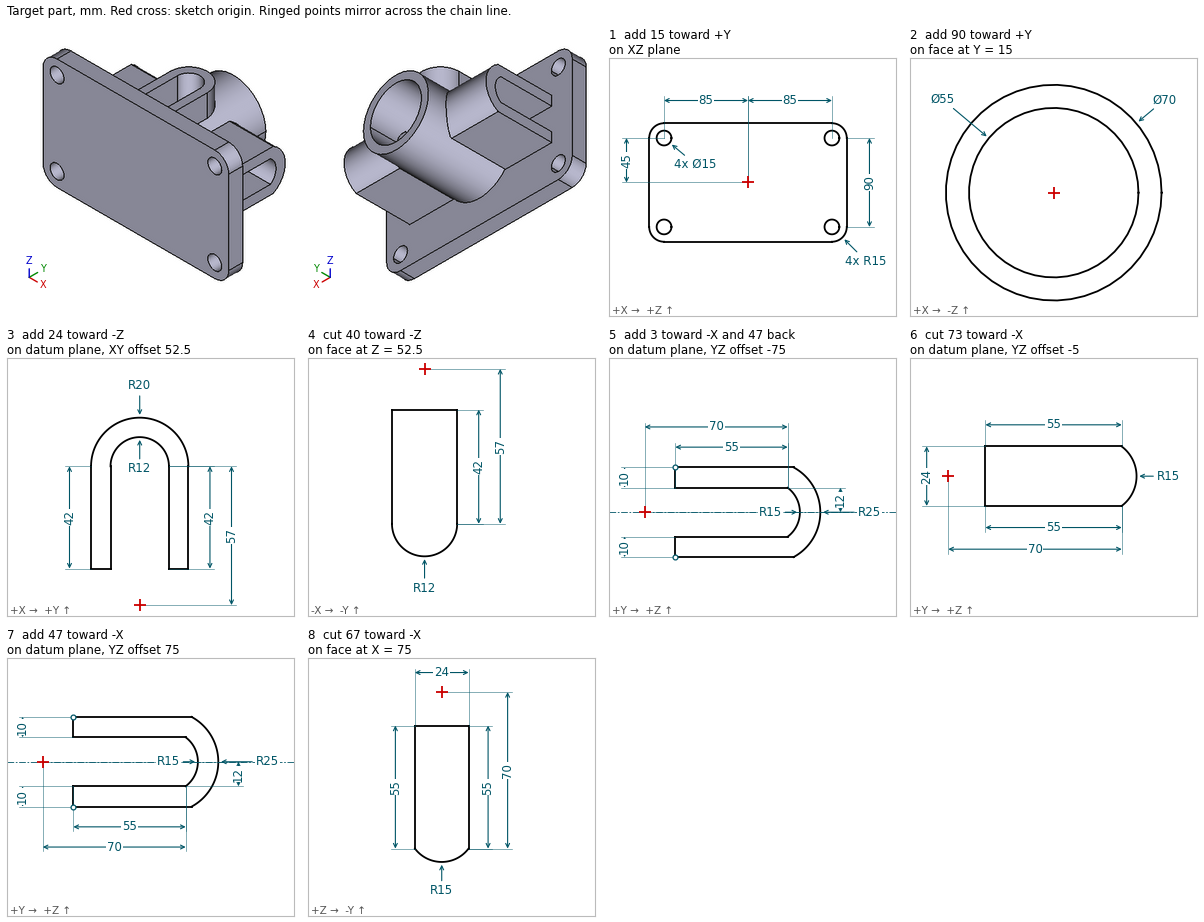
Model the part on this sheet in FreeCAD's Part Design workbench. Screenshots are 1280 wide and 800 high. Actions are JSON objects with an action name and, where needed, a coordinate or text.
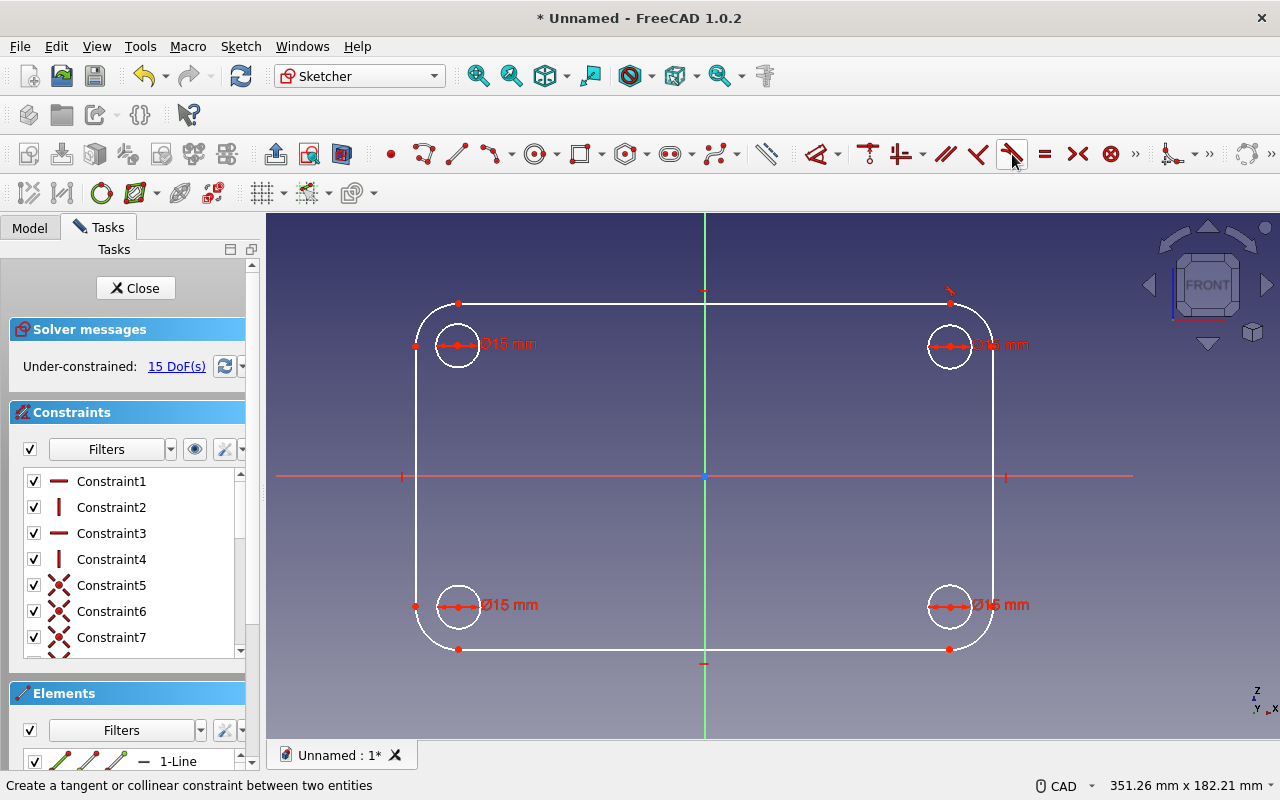
{"action": "left_click", "coordinate": [606, 304]}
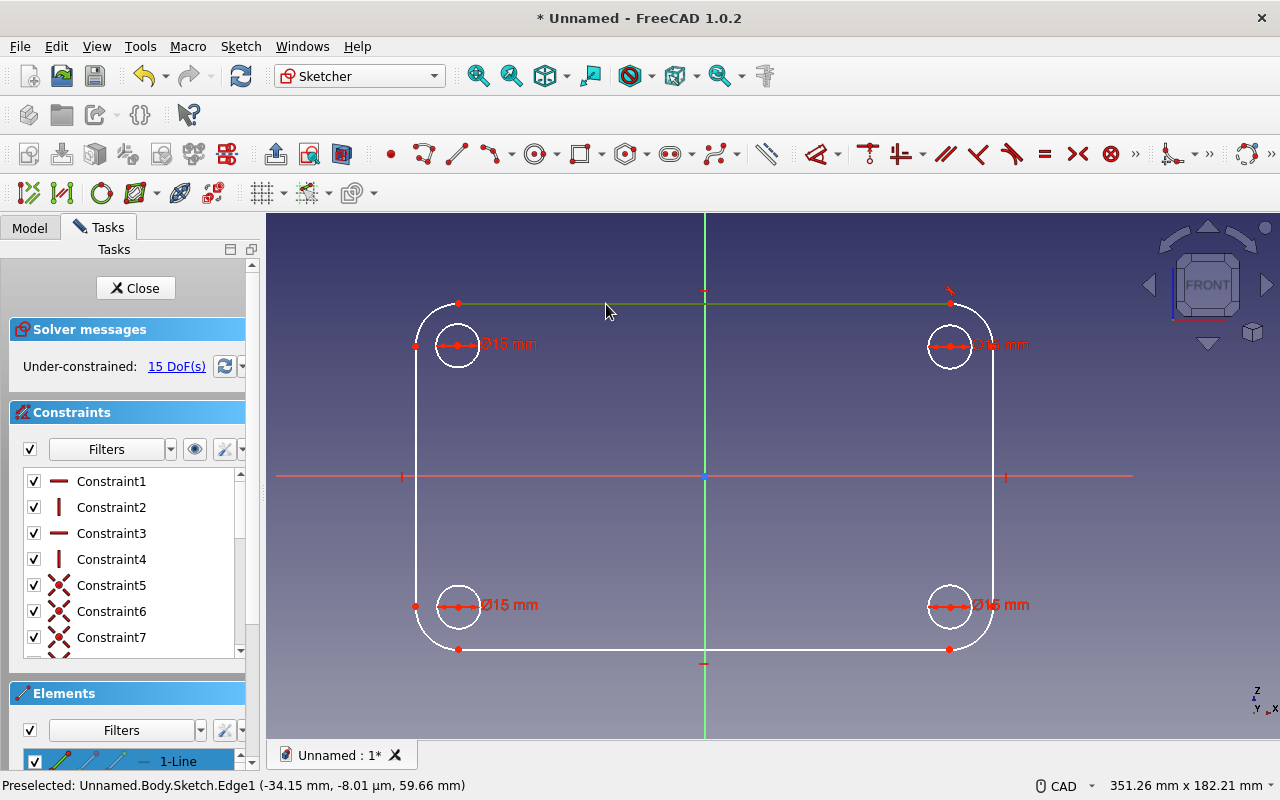
{"action": "left_click", "coordinate": [439, 308]}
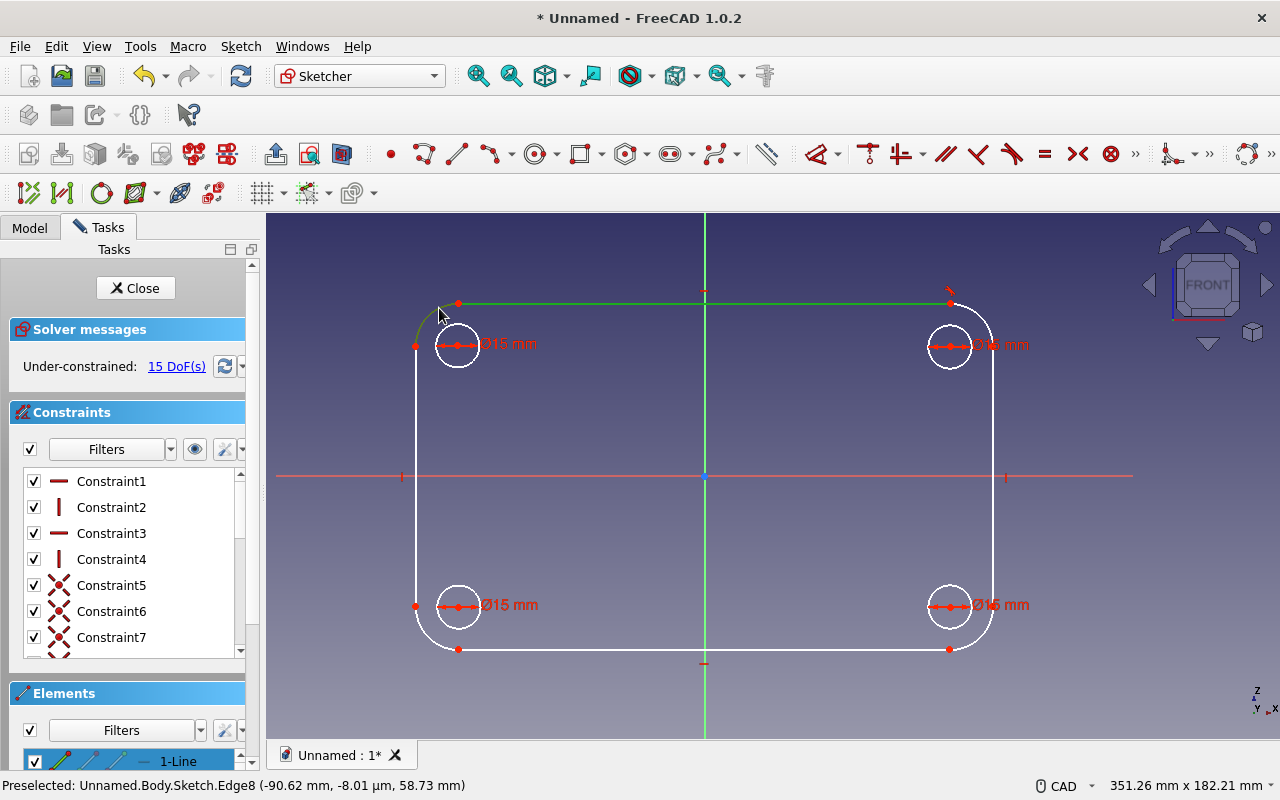
{"action": "left_click", "coordinate": [1012, 154]}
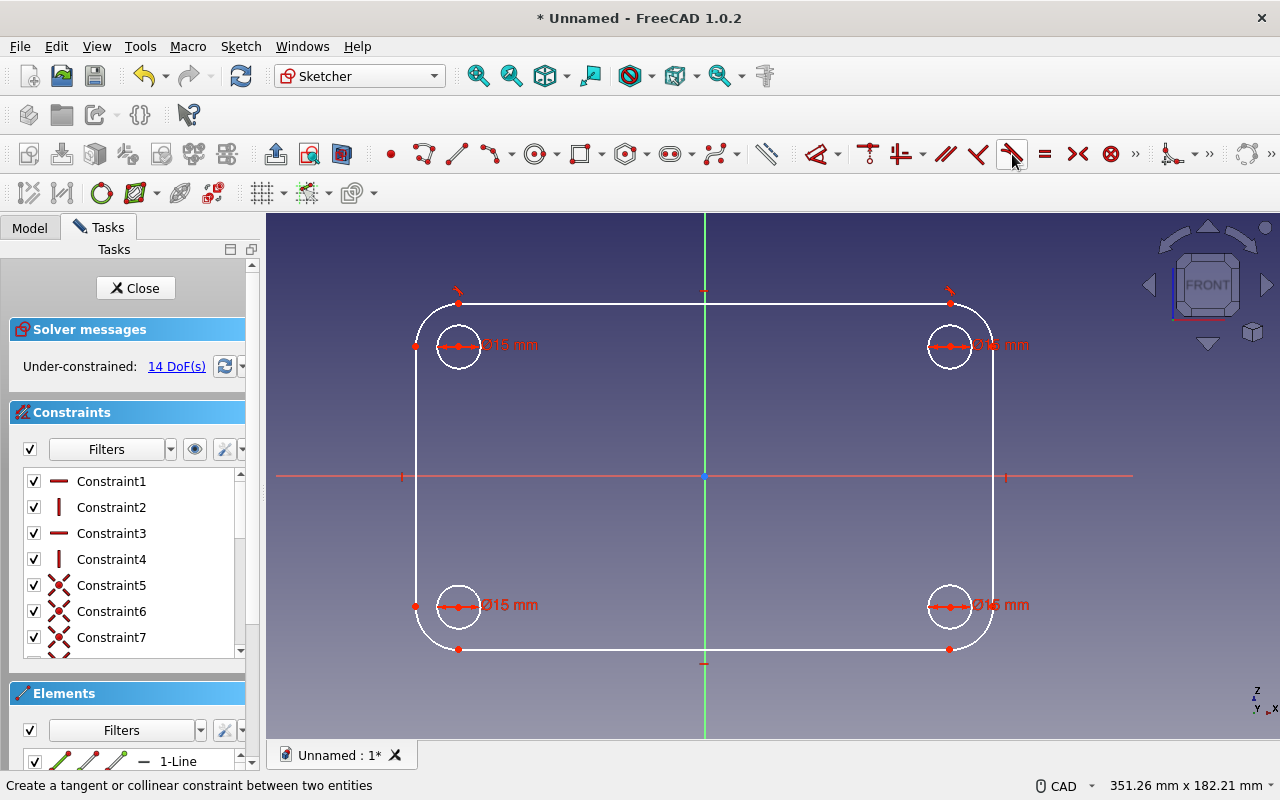
{"action": "left_click", "coordinate": [993, 425]}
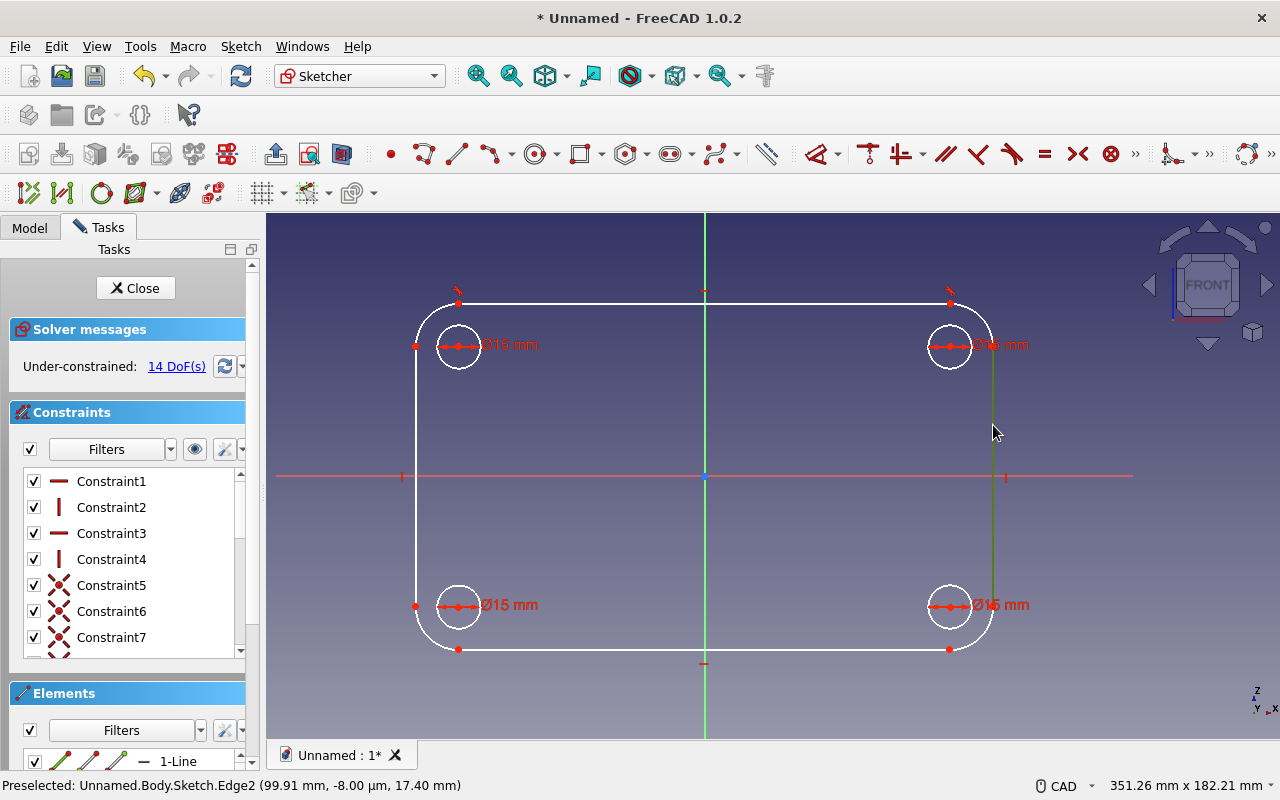
{"action": "left_click", "coordinate": [988, 327]}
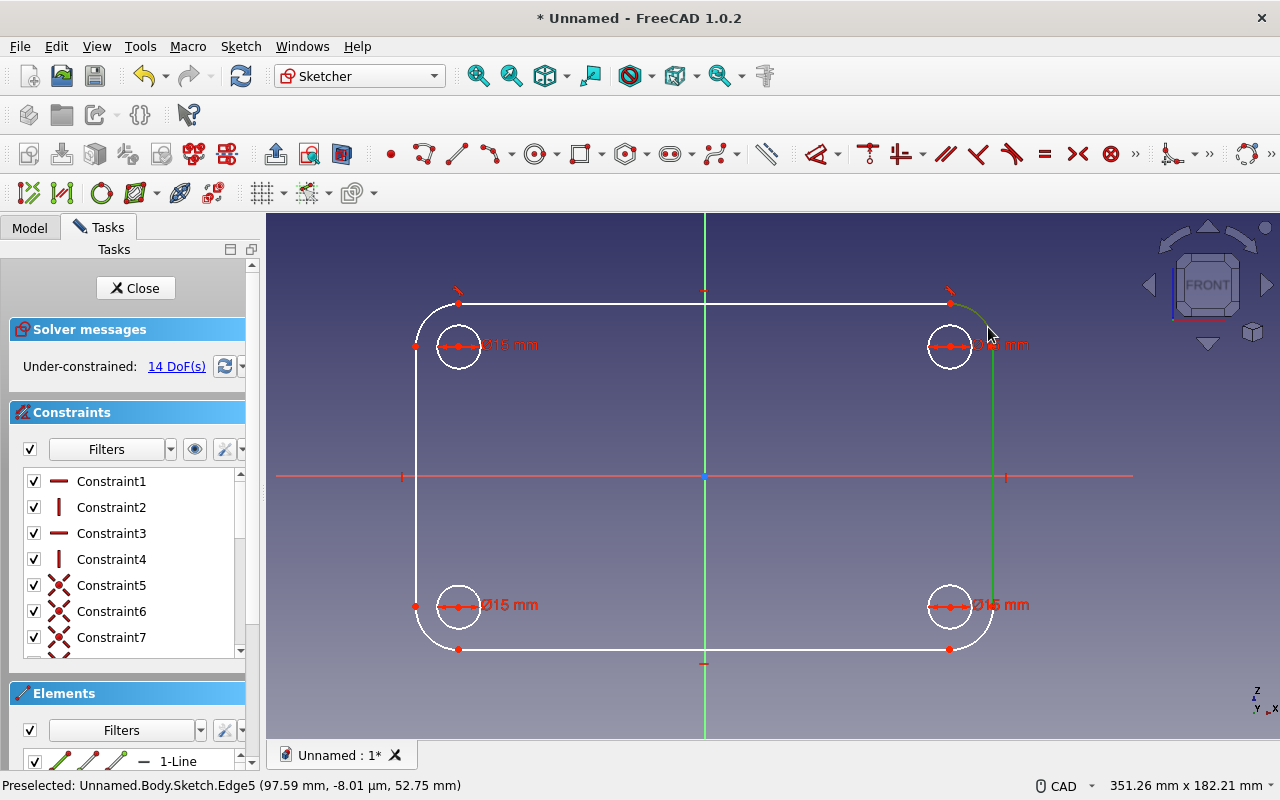
{"action": "key", "text": "t"}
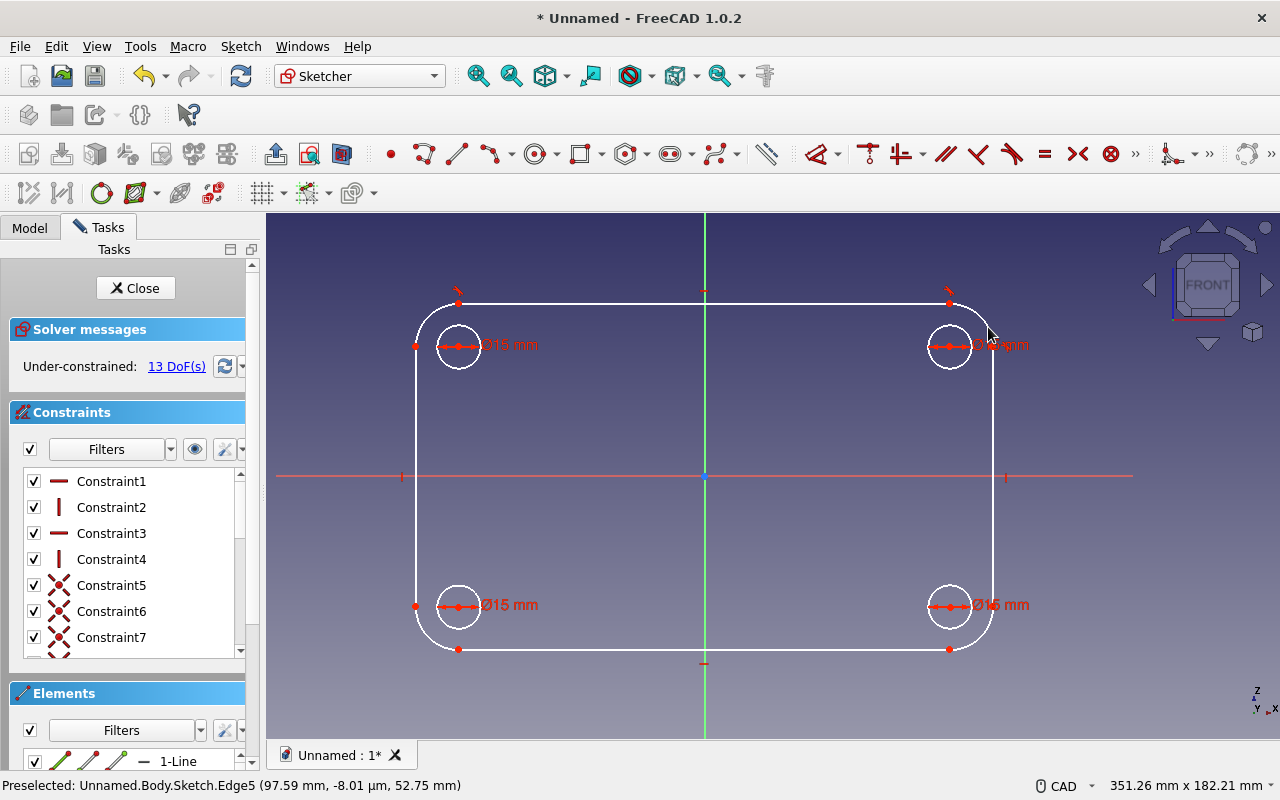
{"action": "left_click", "coordinate": [993, 425]}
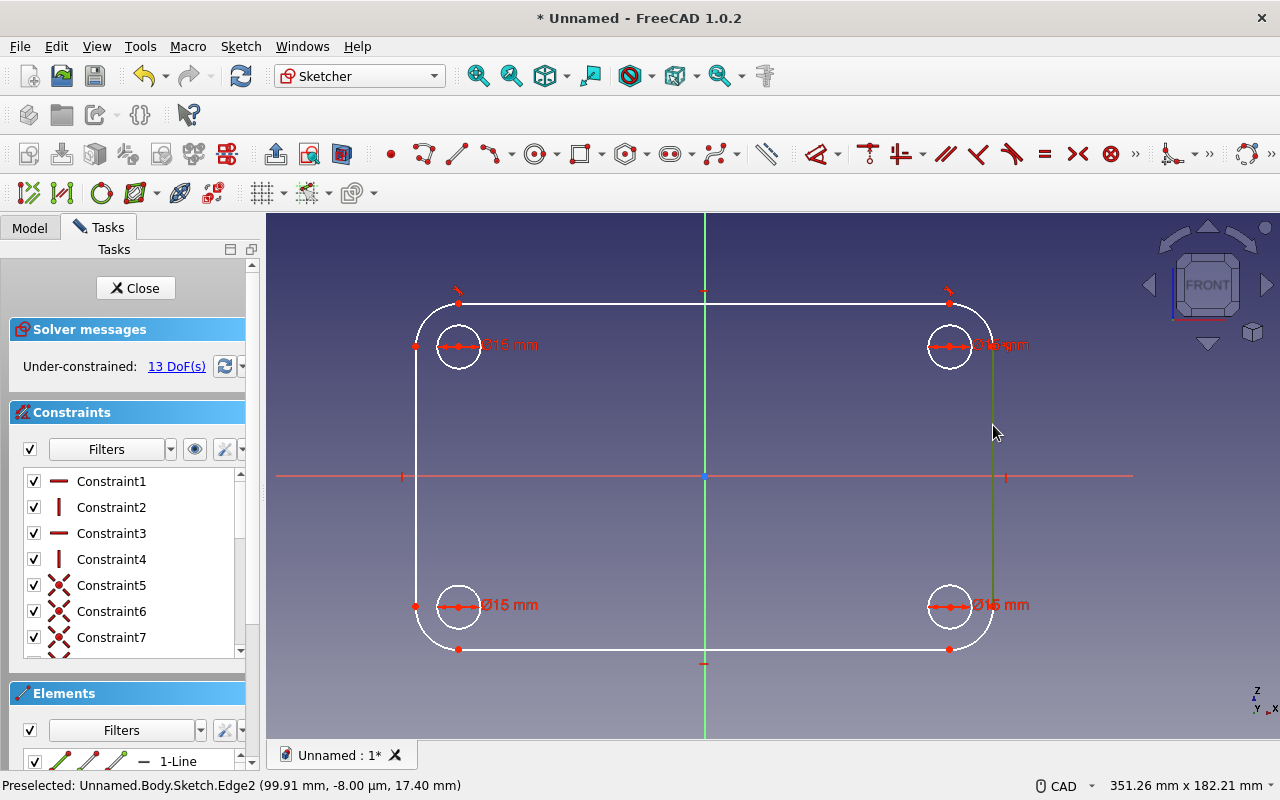
{"action": "left_click", "coordinate": [970, 645]}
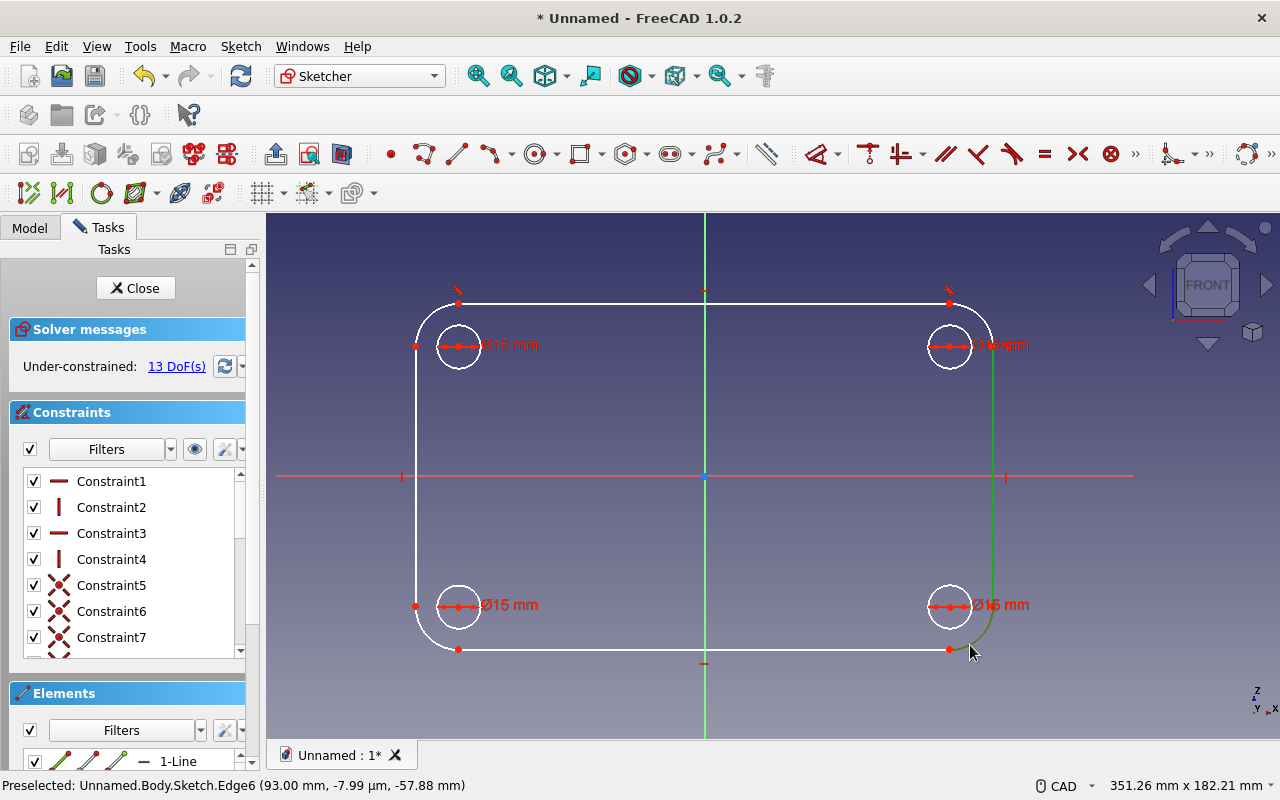
{"action": "key", "text": "t"}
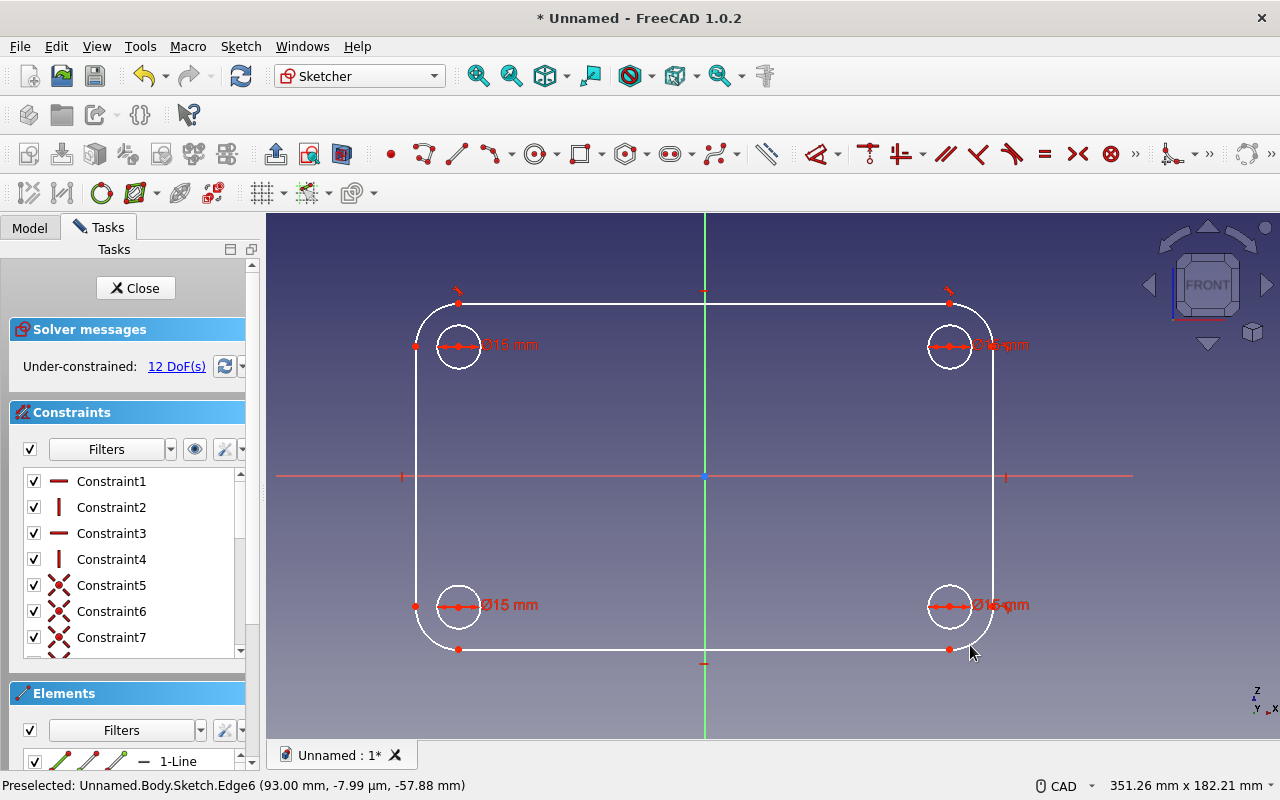
{"action": "left_click", "coordinate": [803, 650]}